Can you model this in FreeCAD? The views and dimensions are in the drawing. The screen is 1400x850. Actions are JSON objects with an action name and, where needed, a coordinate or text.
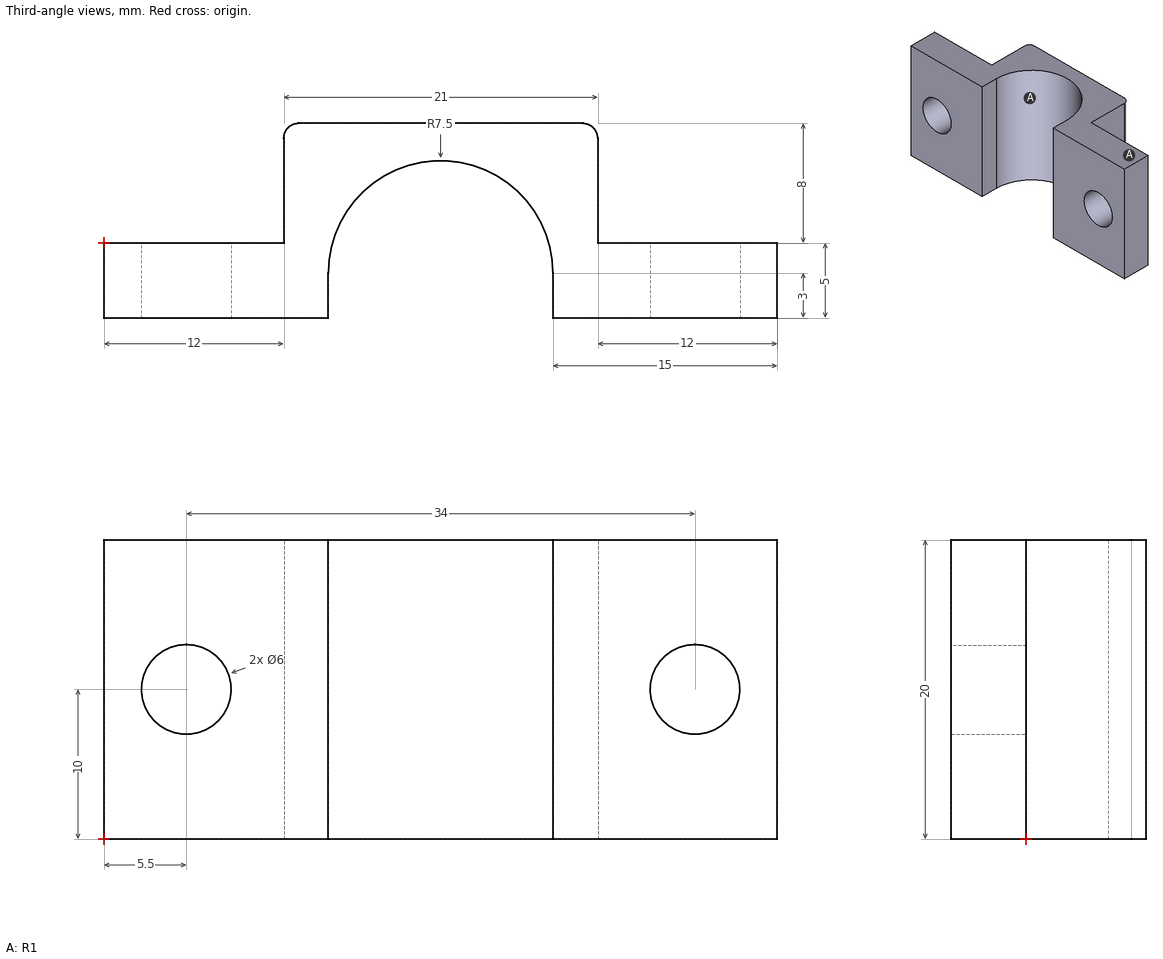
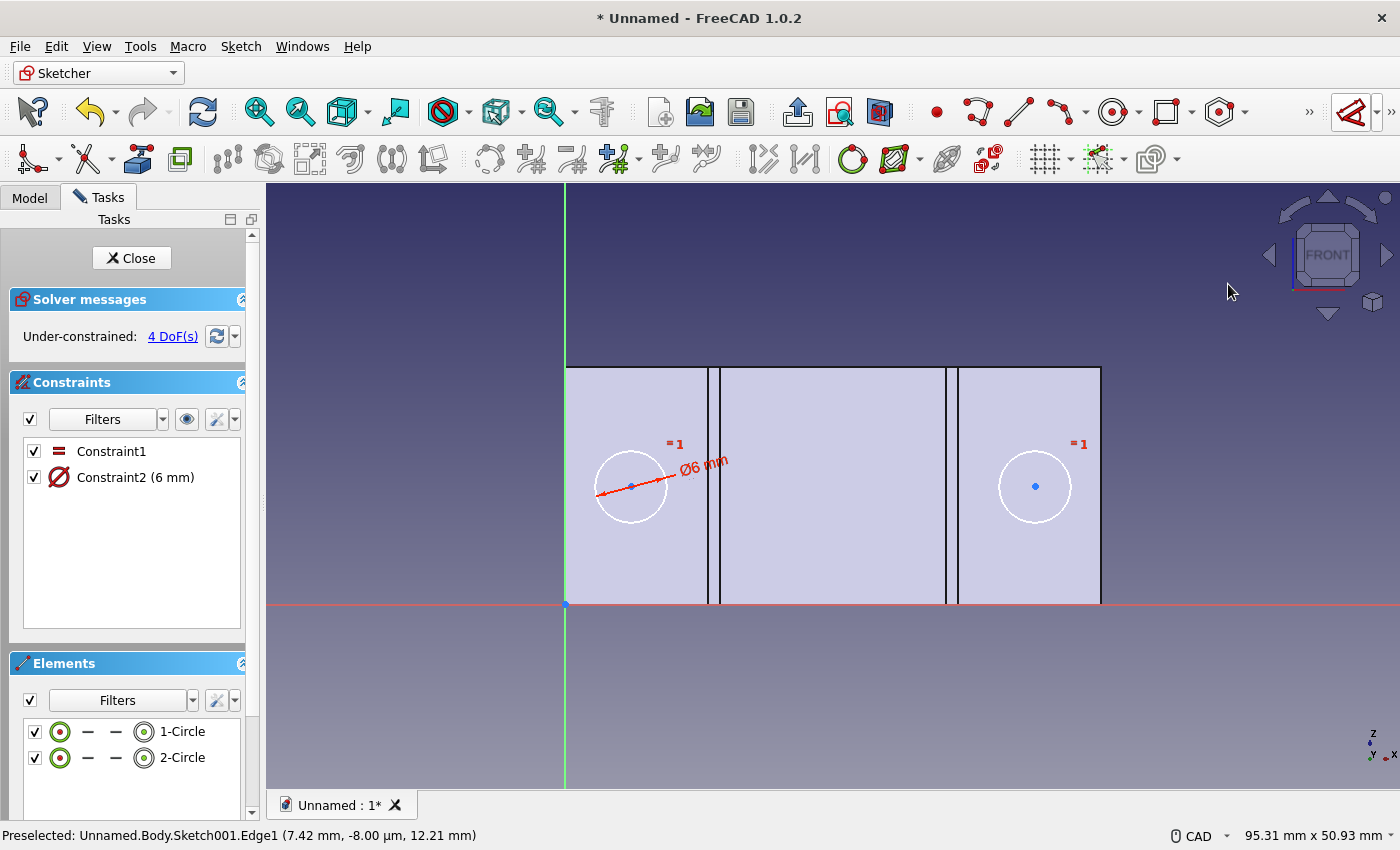
{"action": "left_click", "coordinate": [631, 487]}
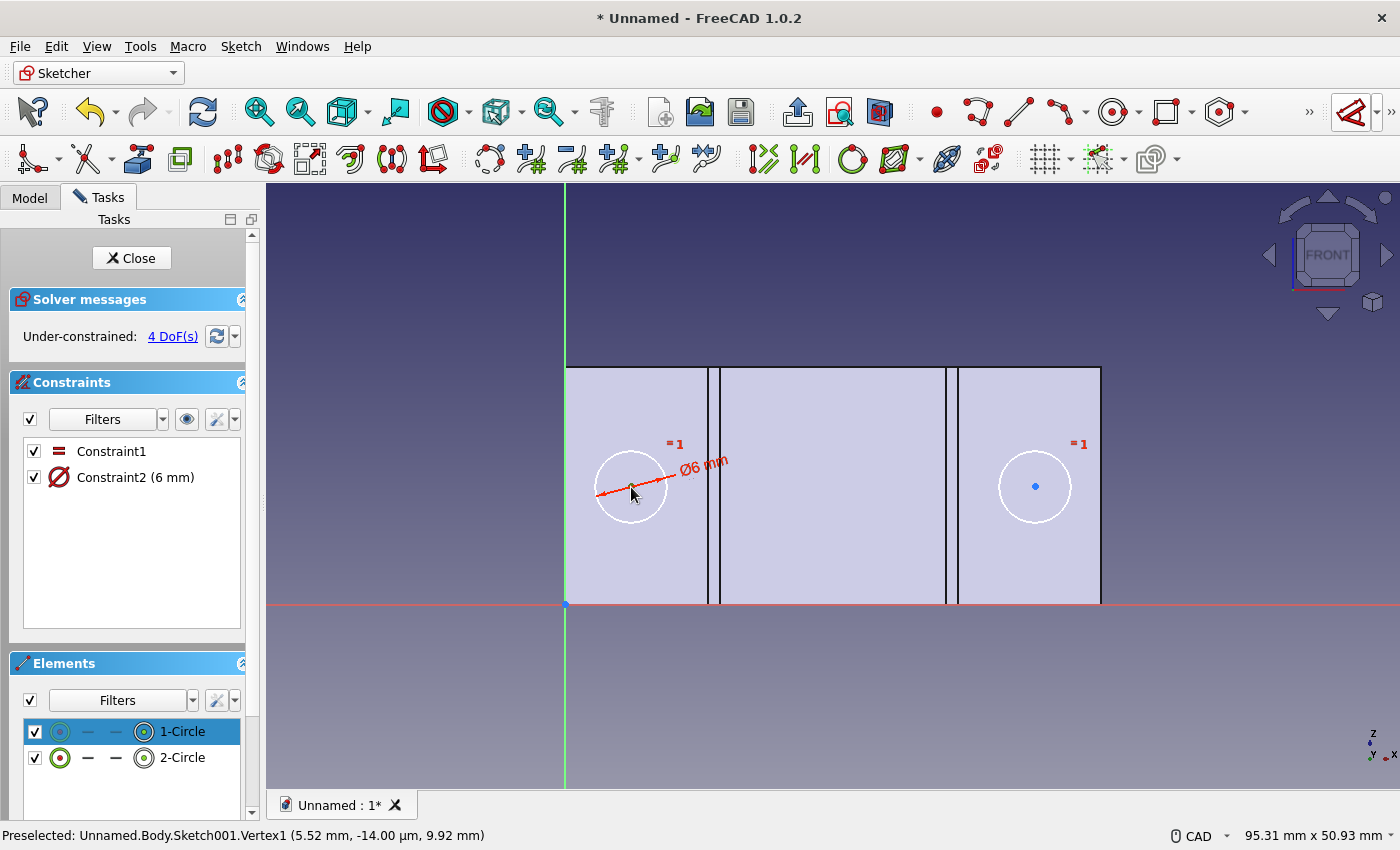
{"action": "key", "text": "i"}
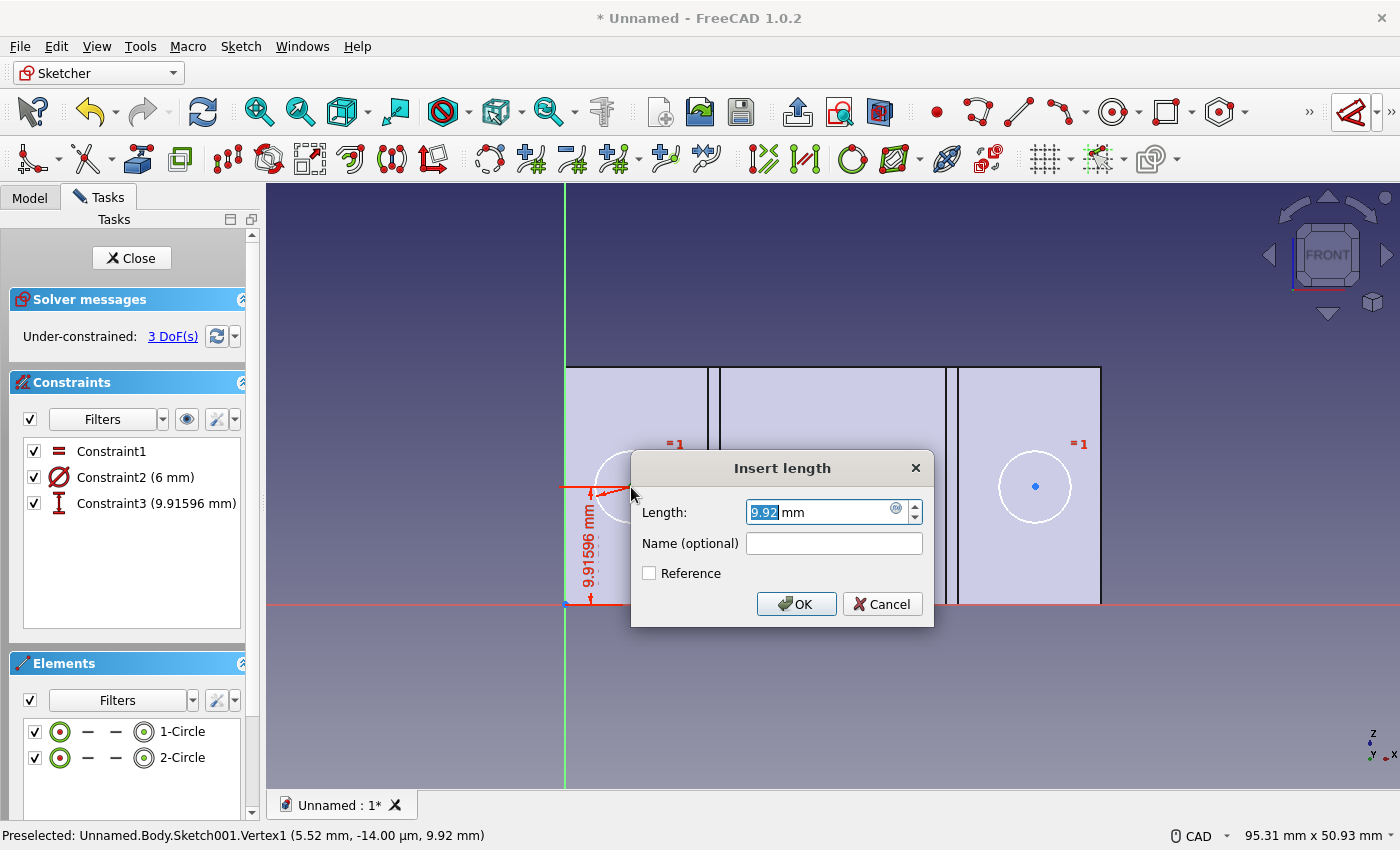
{"action": "type", "text": "10"}
{"action": "key", "text": "Return"}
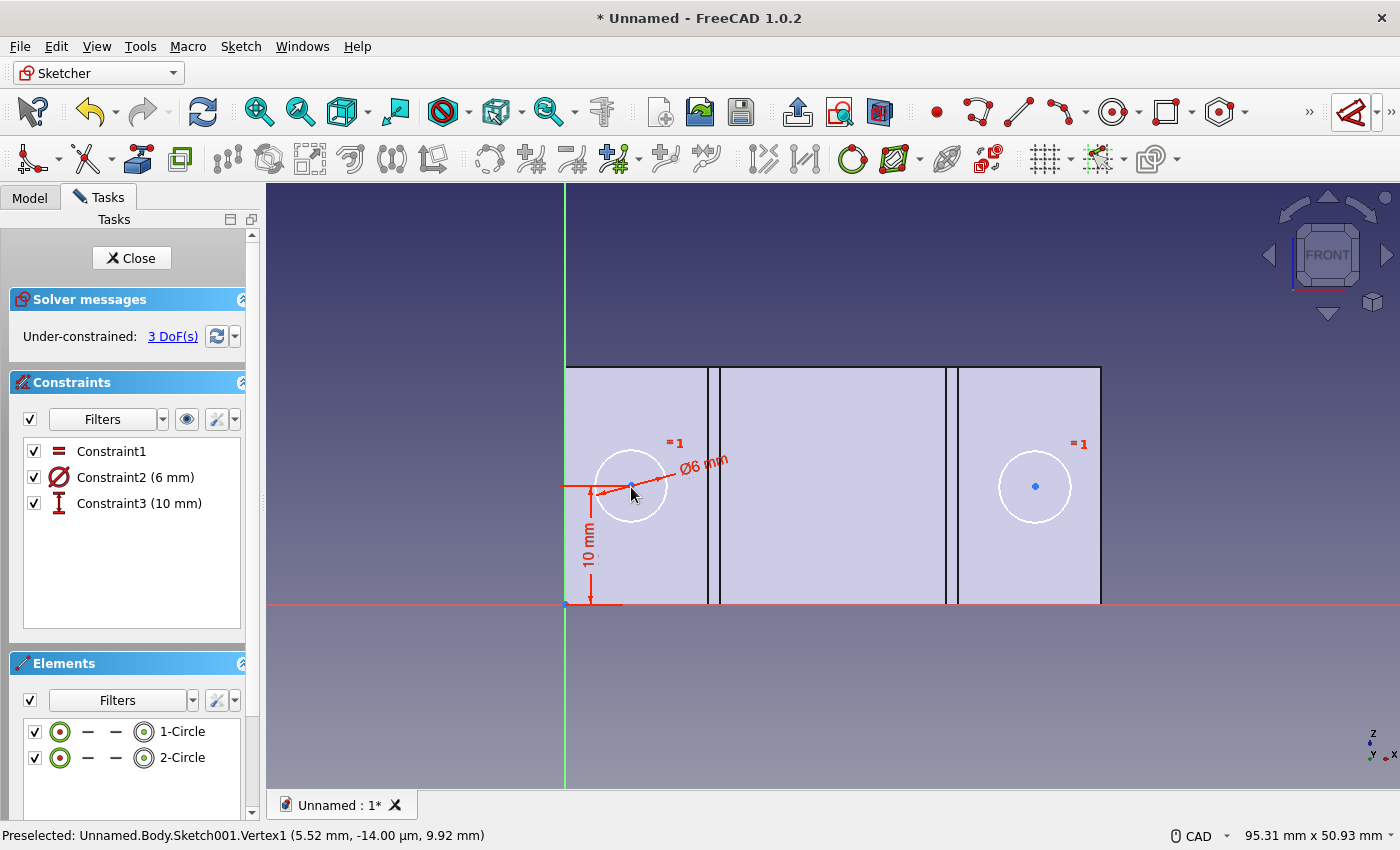
{"action": "left_click", "coordinate": [1035, 487]}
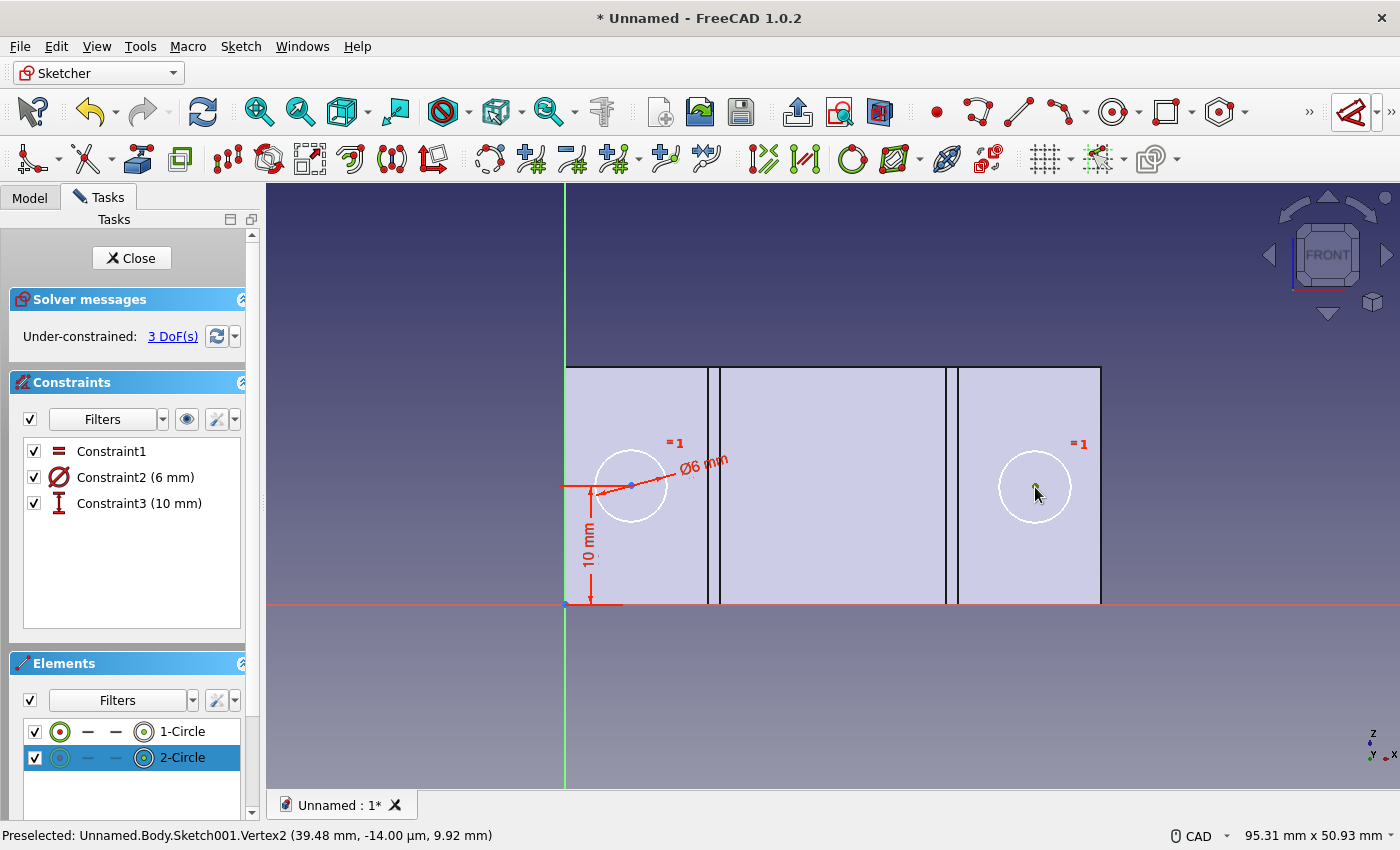
{"action": "key", "text": "i"}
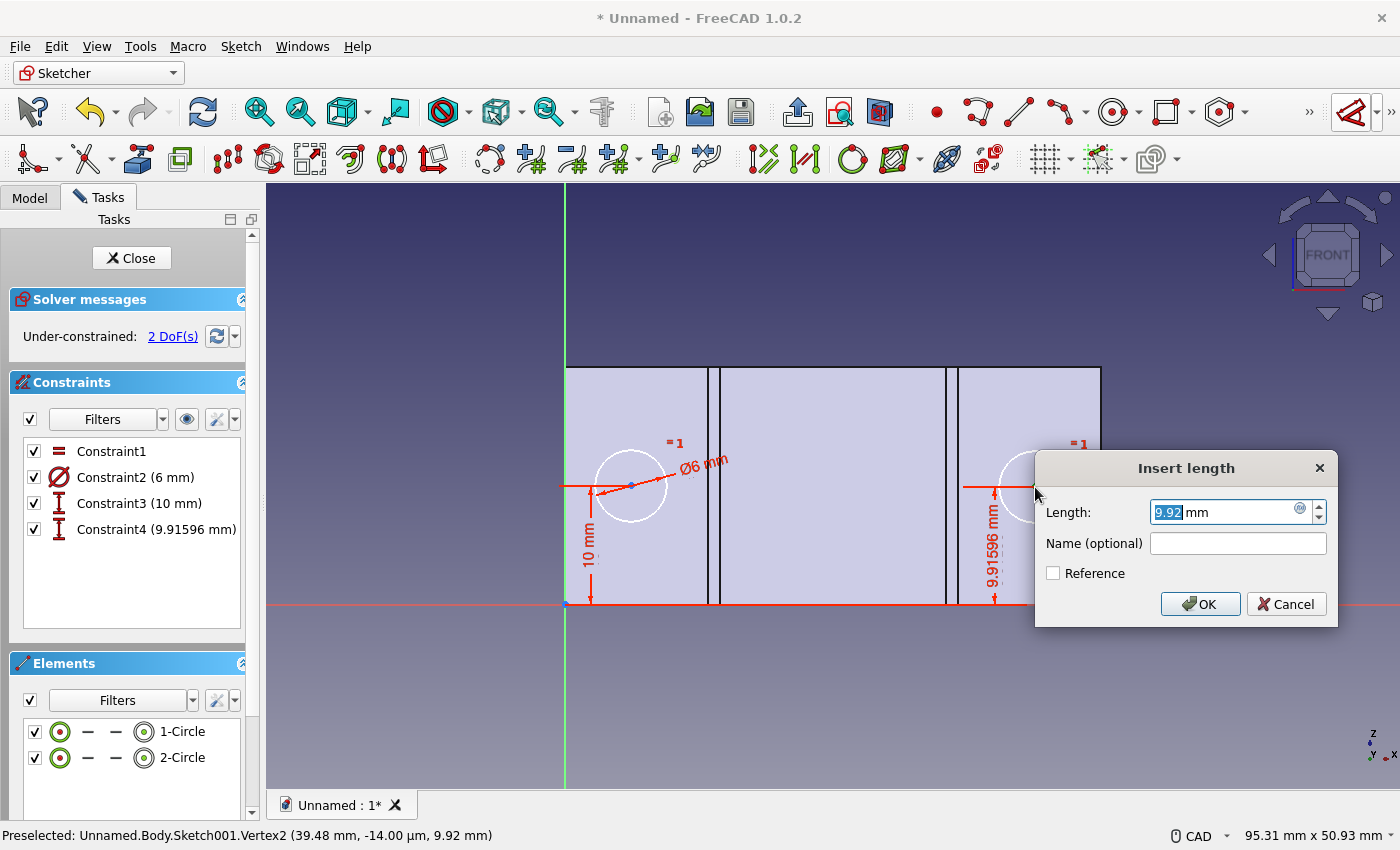
{"action": "type", "text": "10"}
{"action": "key", "text": "Return"}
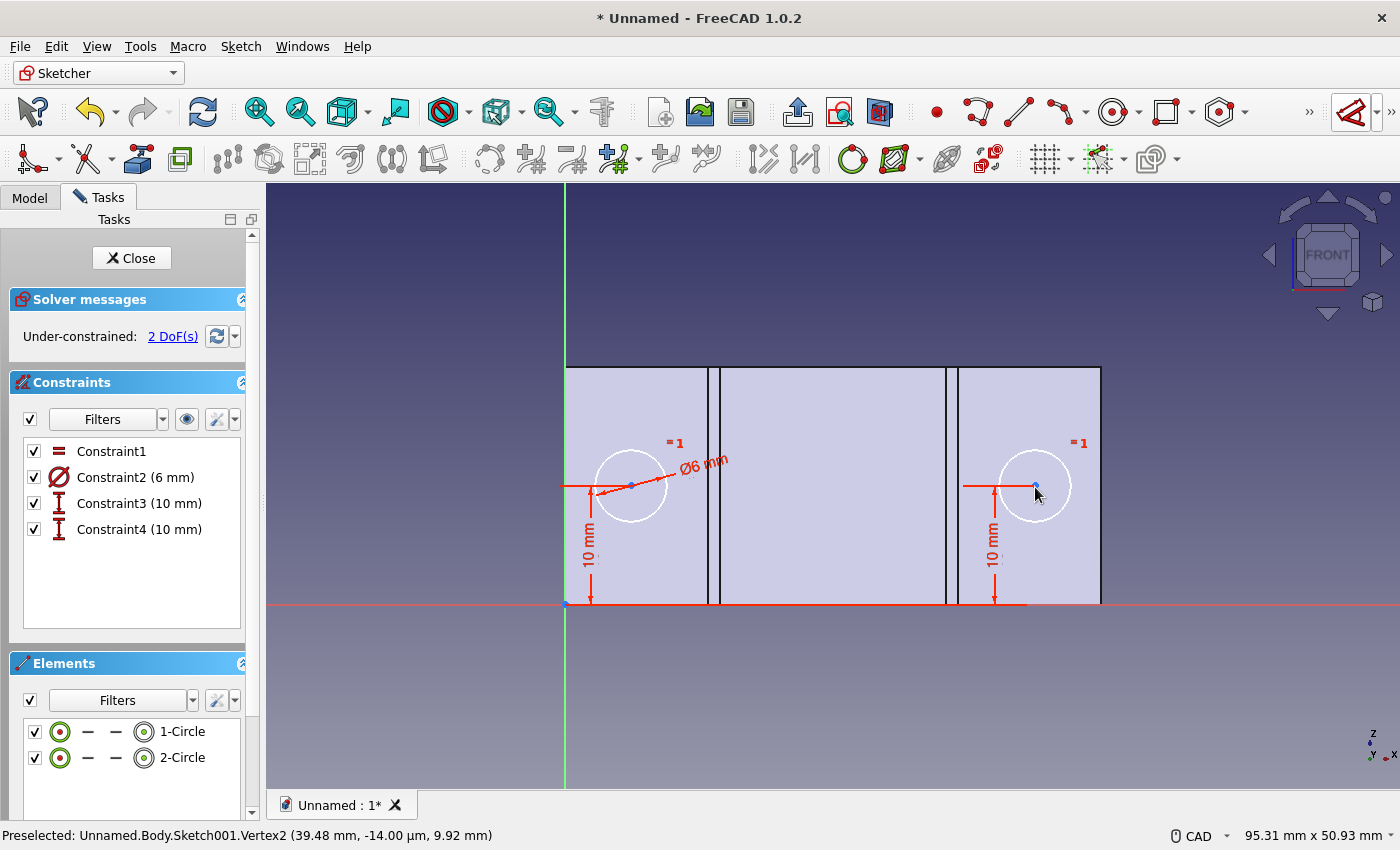
{"action": "left_click", "coordinate": [631, 486]}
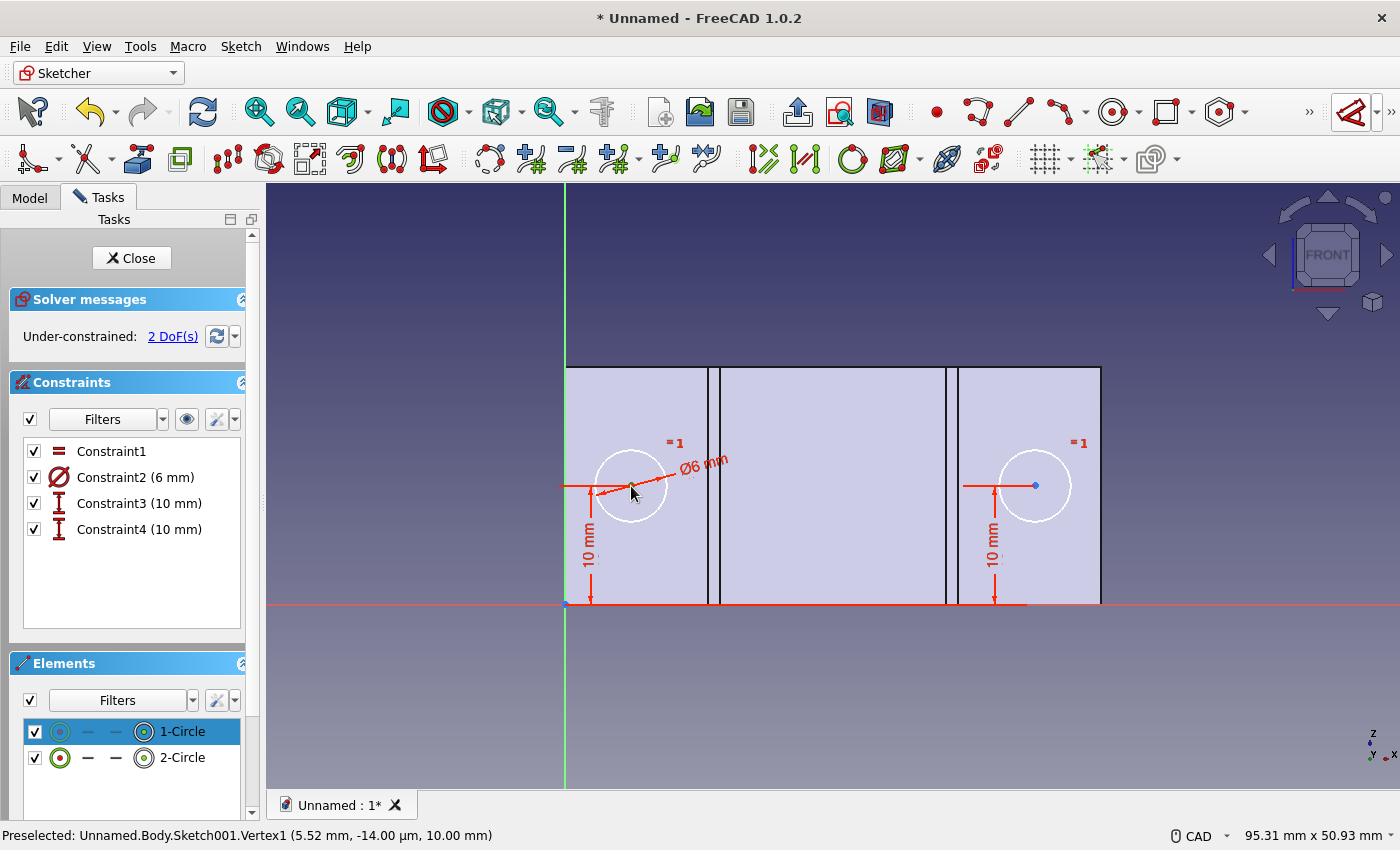
{"action": "key", "text": "l"}